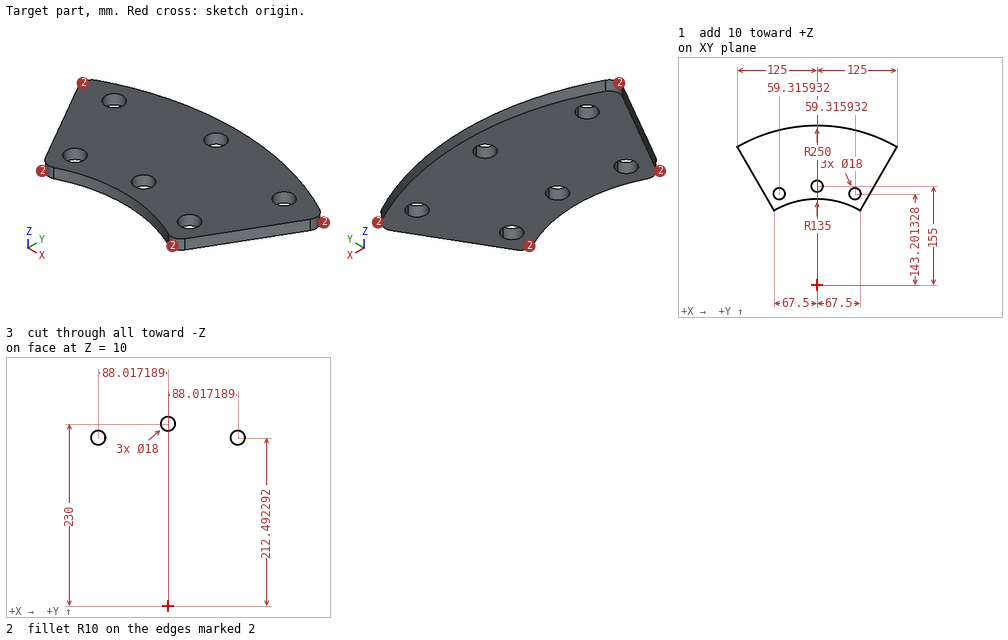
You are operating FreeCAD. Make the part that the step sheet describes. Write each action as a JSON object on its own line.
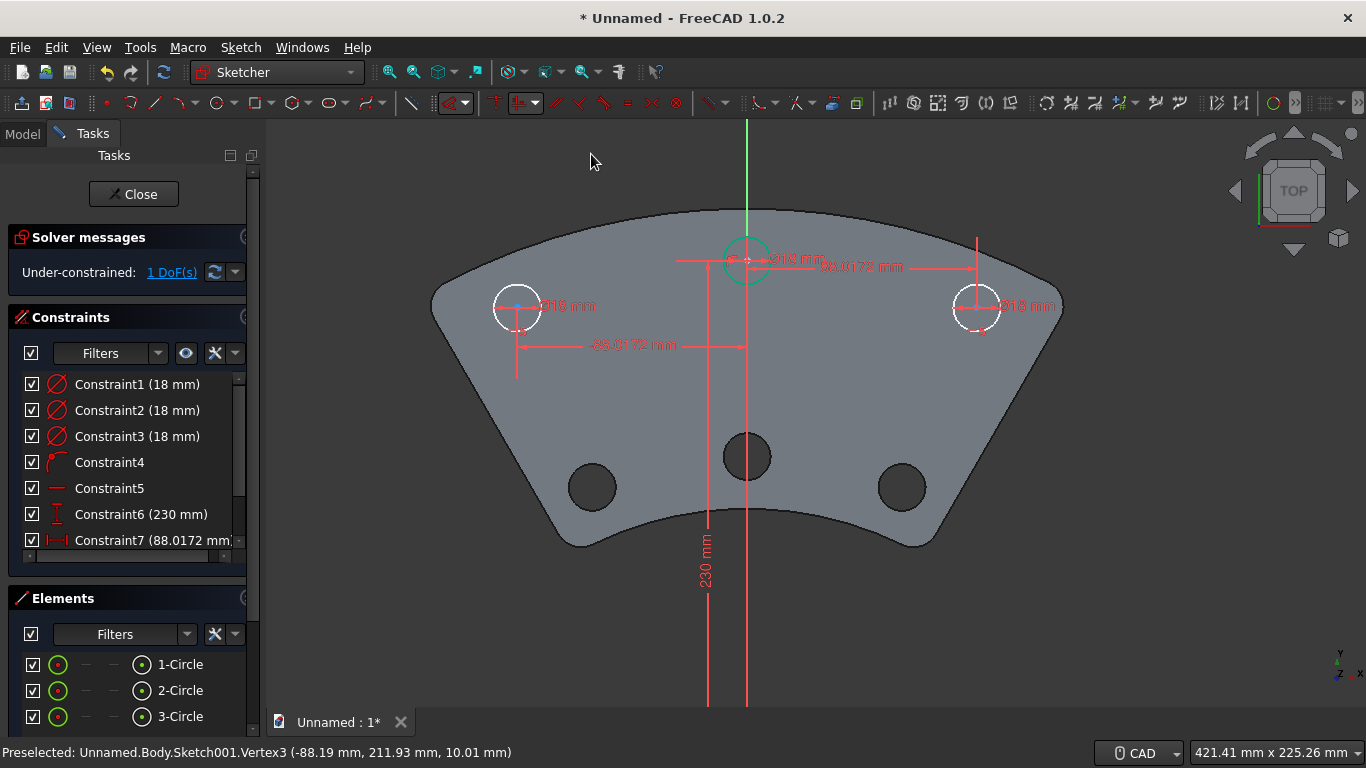
{"action": "left_click", "coordinate": [977, 308]}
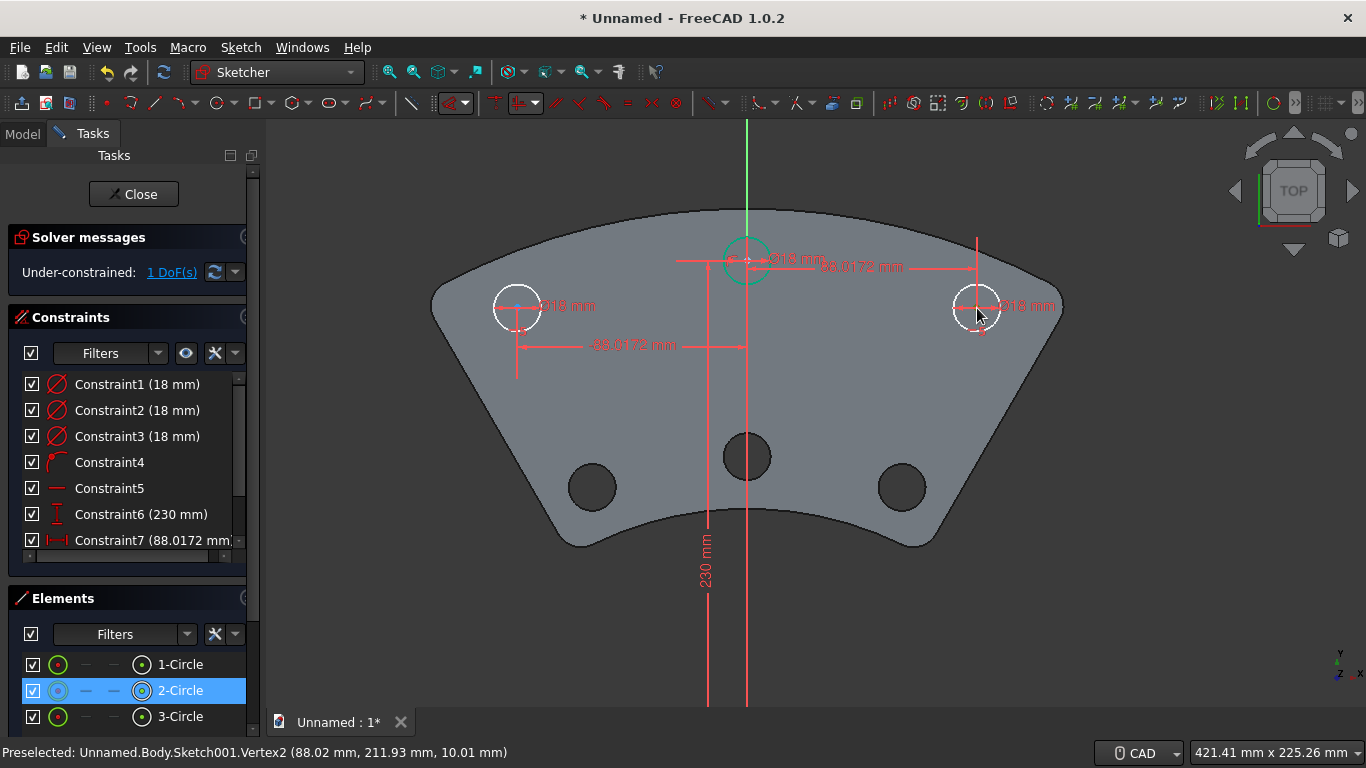
{"action": "key", "text": "i"}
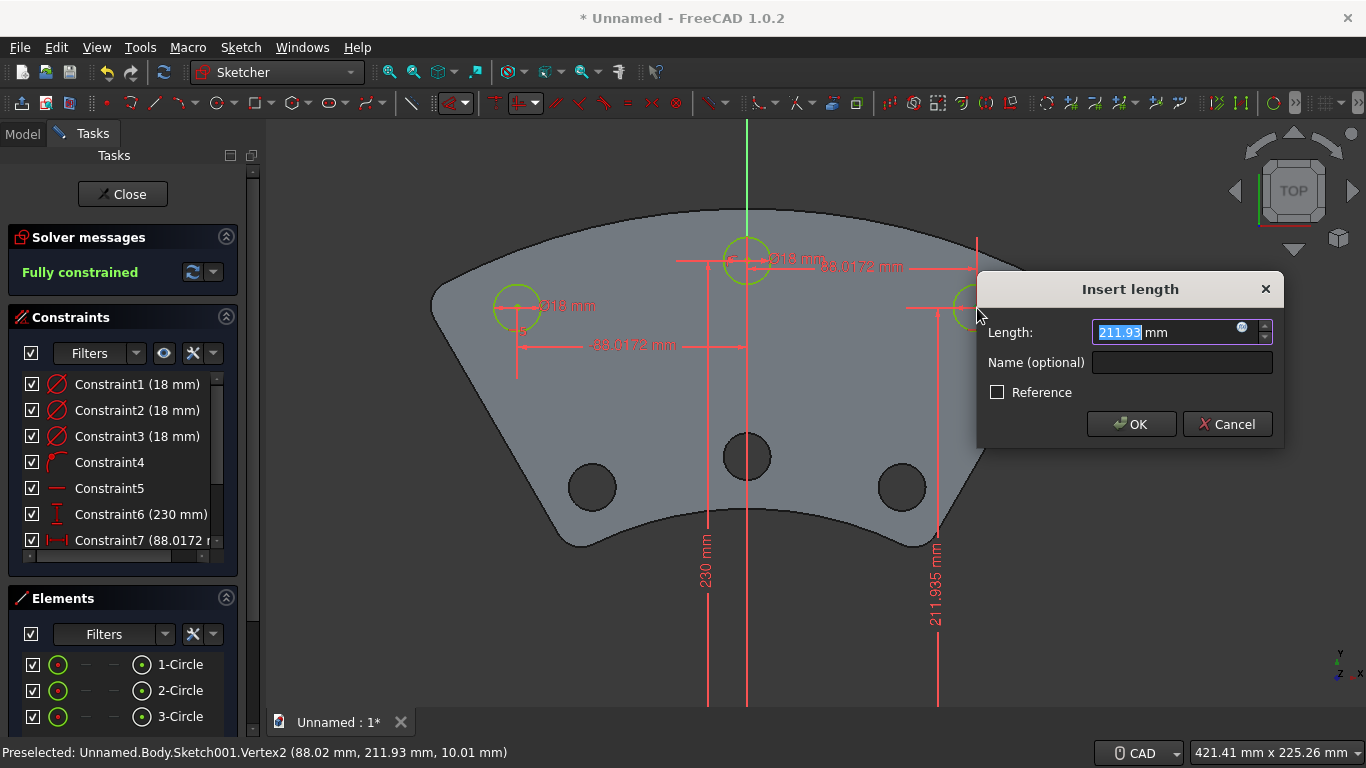
{"action": "type", "text": "212.492292"}
{"action": "key", "text": "Return"}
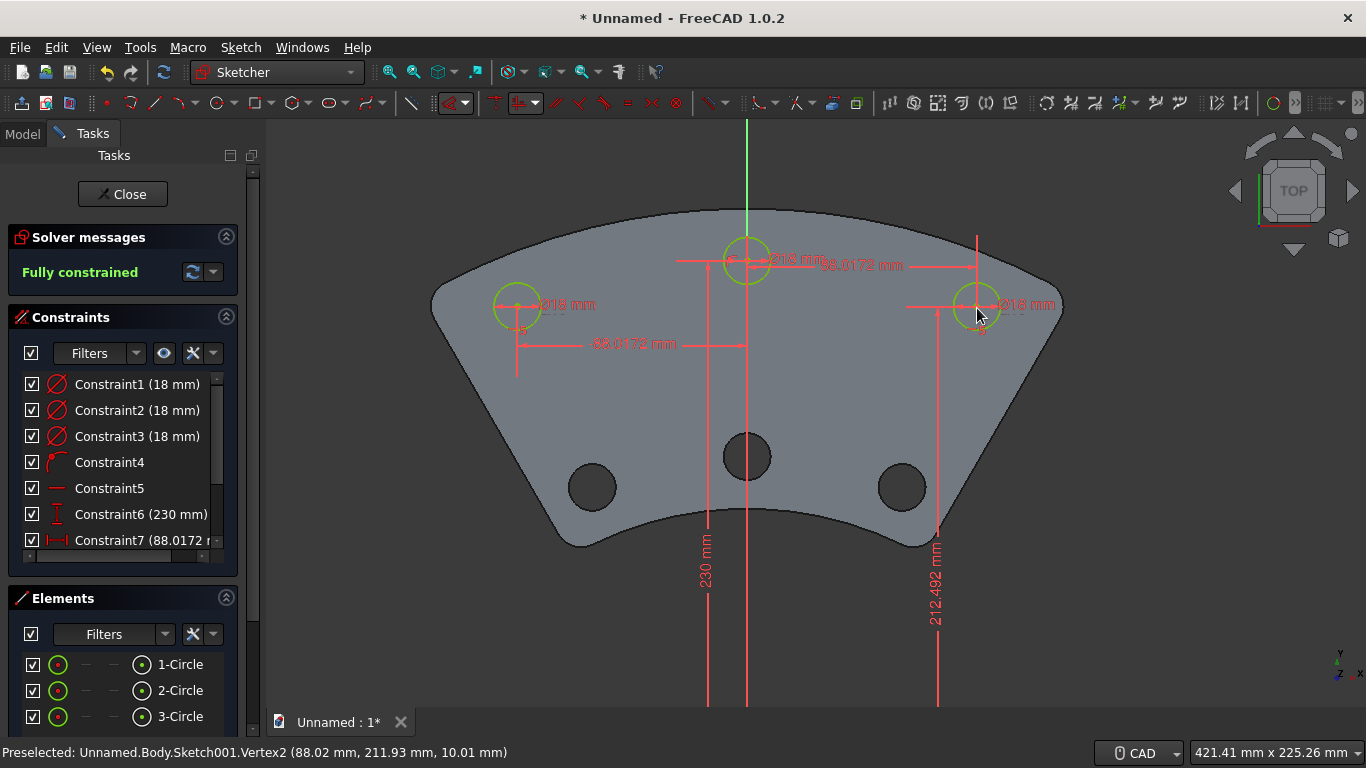
{"action": "left_click", "coordinate": [123, 194]}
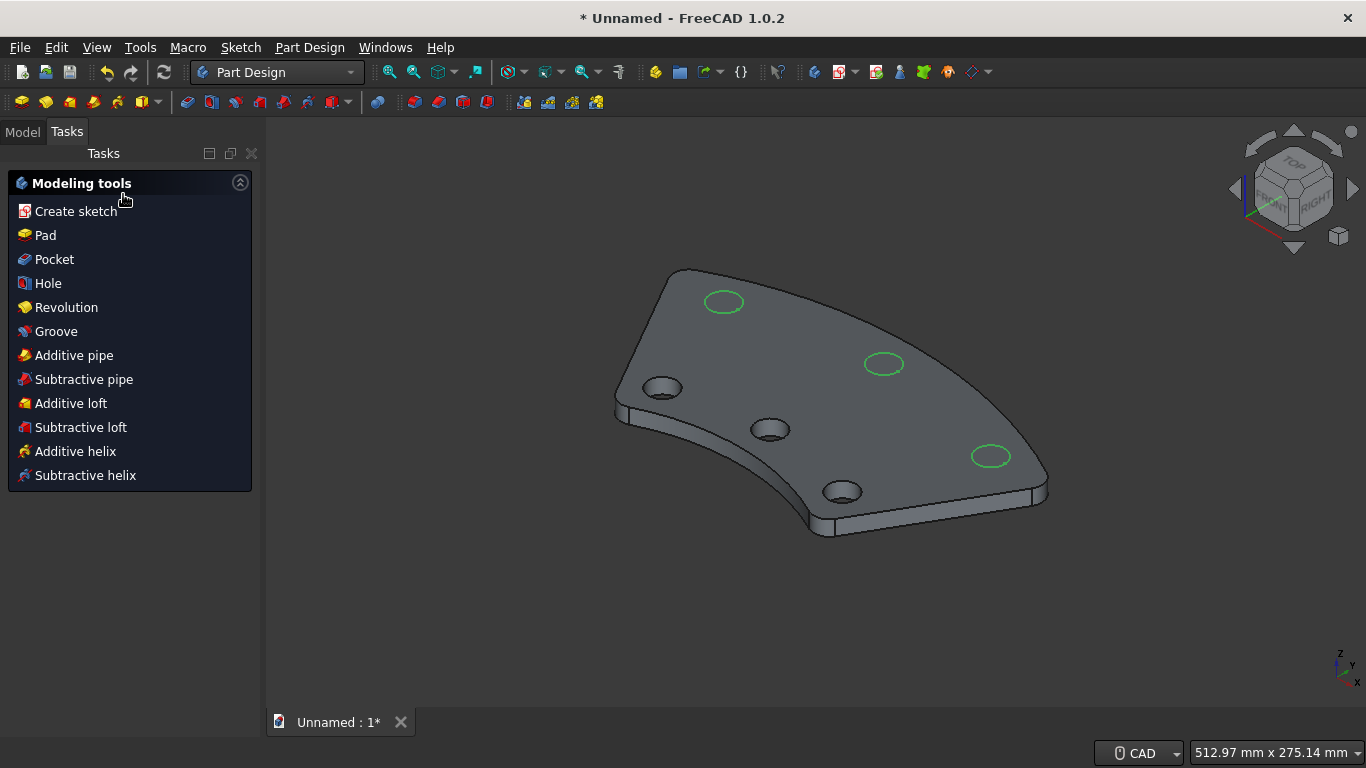
{"action": "left_click", "coordinate": [188, 102]}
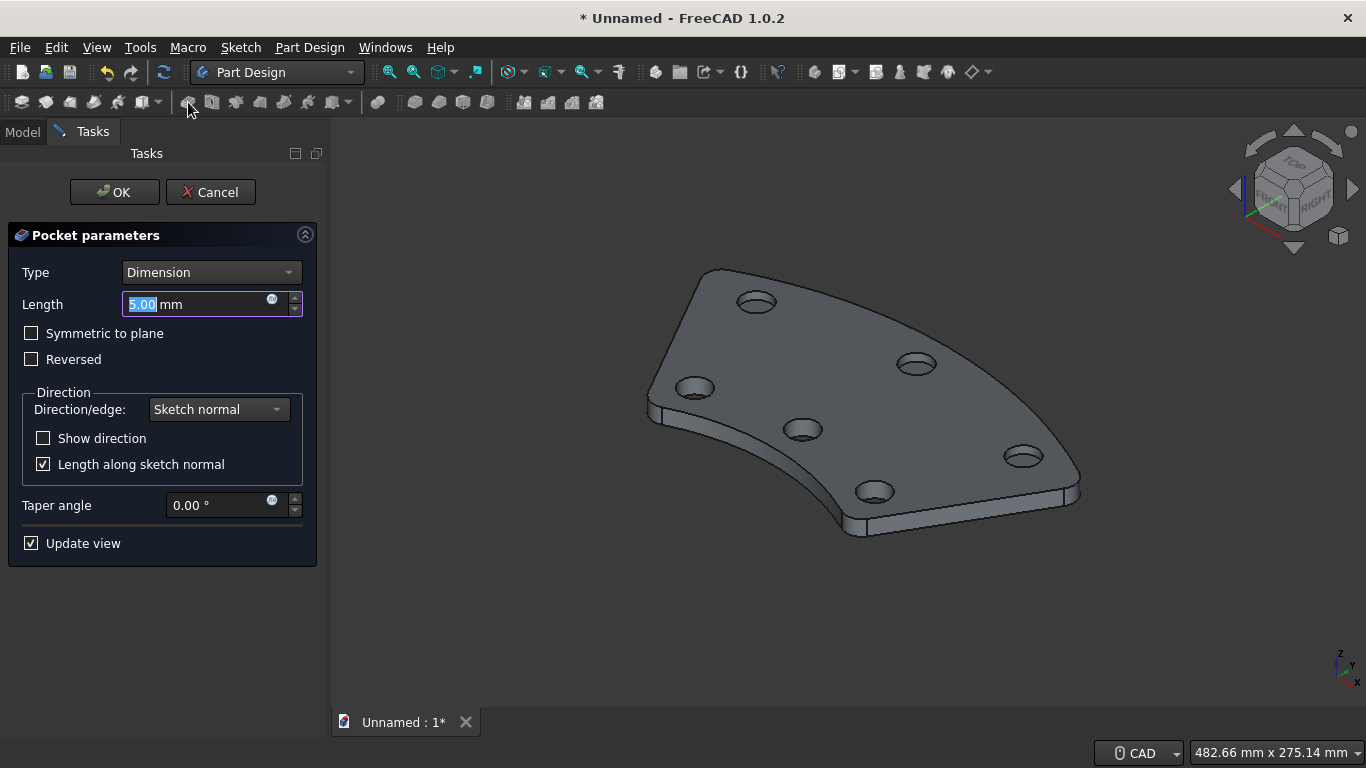
{"action": "left_click", "coordinate": [212, 272]}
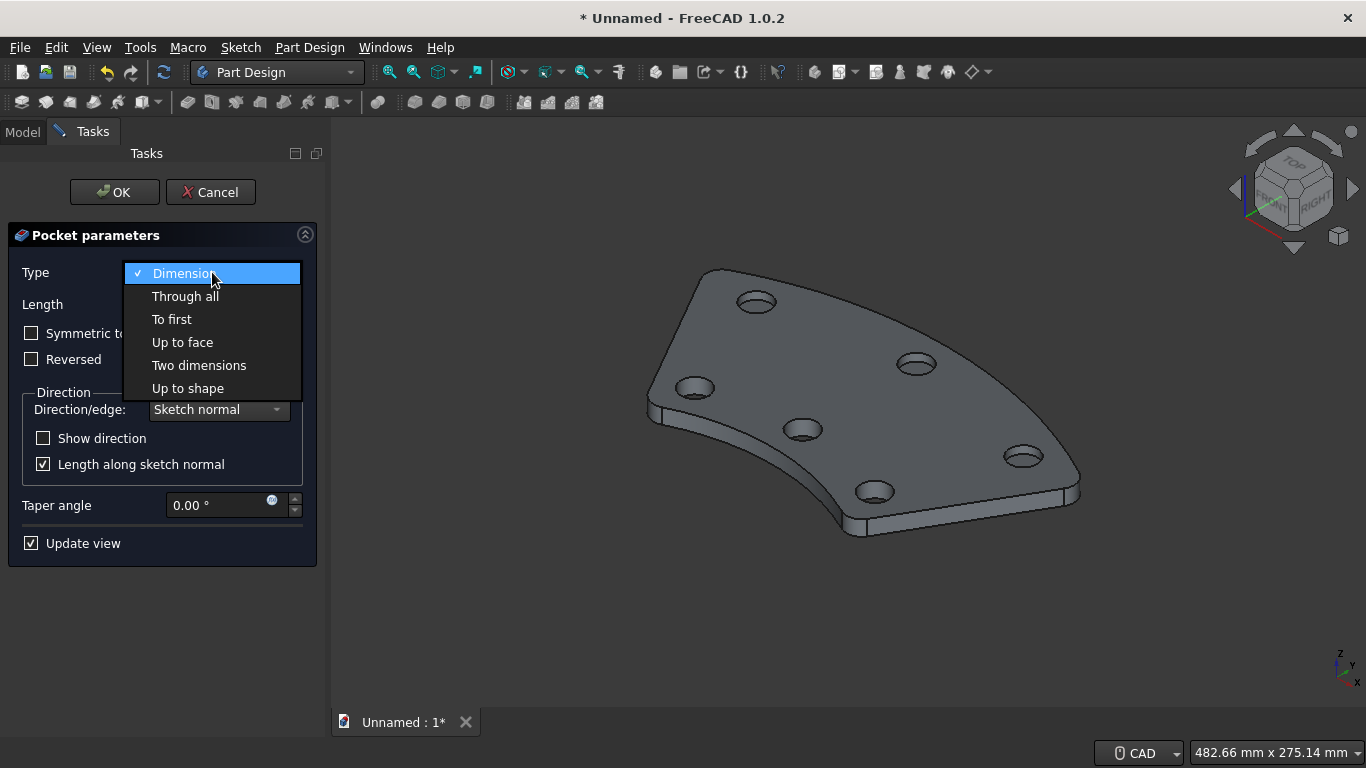
{"action": "left_click", "coordinate": [212, 296]}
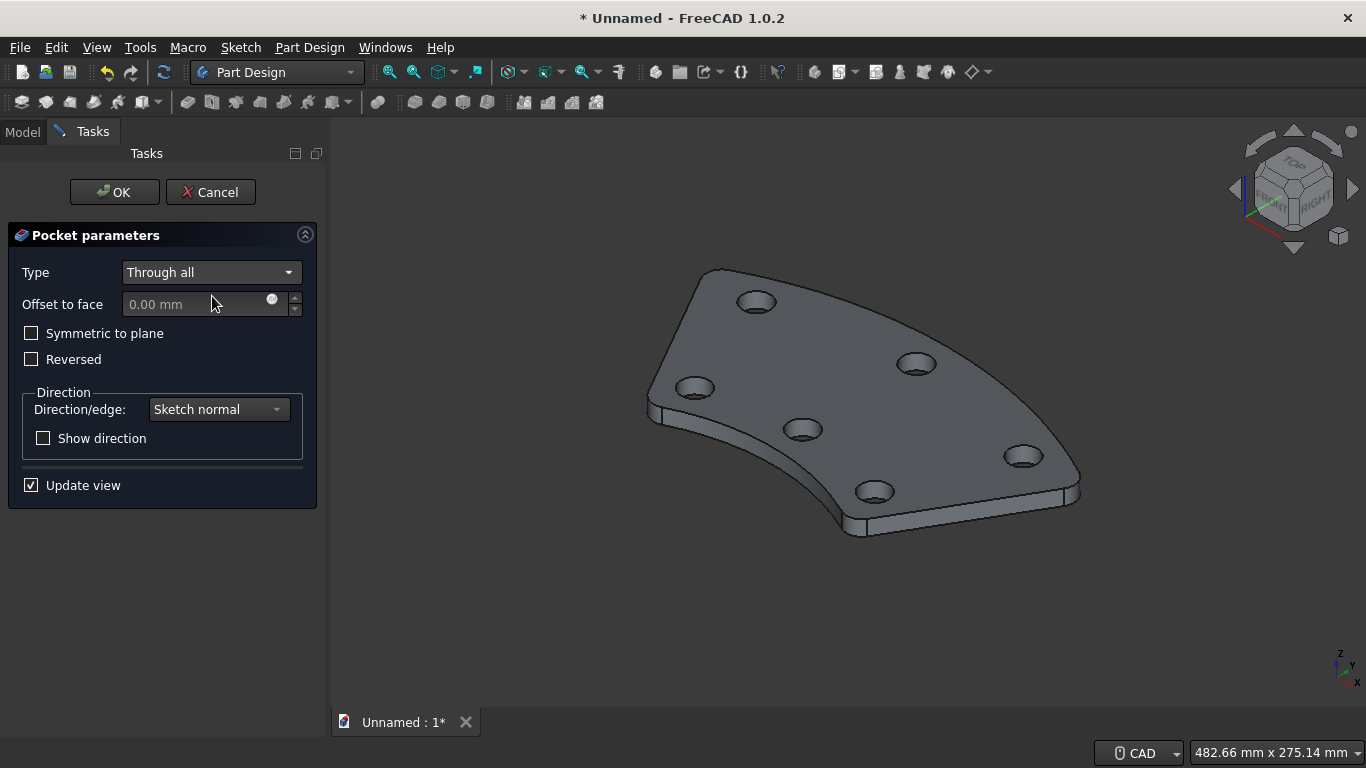
{"action": "left_click", "coordinate": [115, 192]}